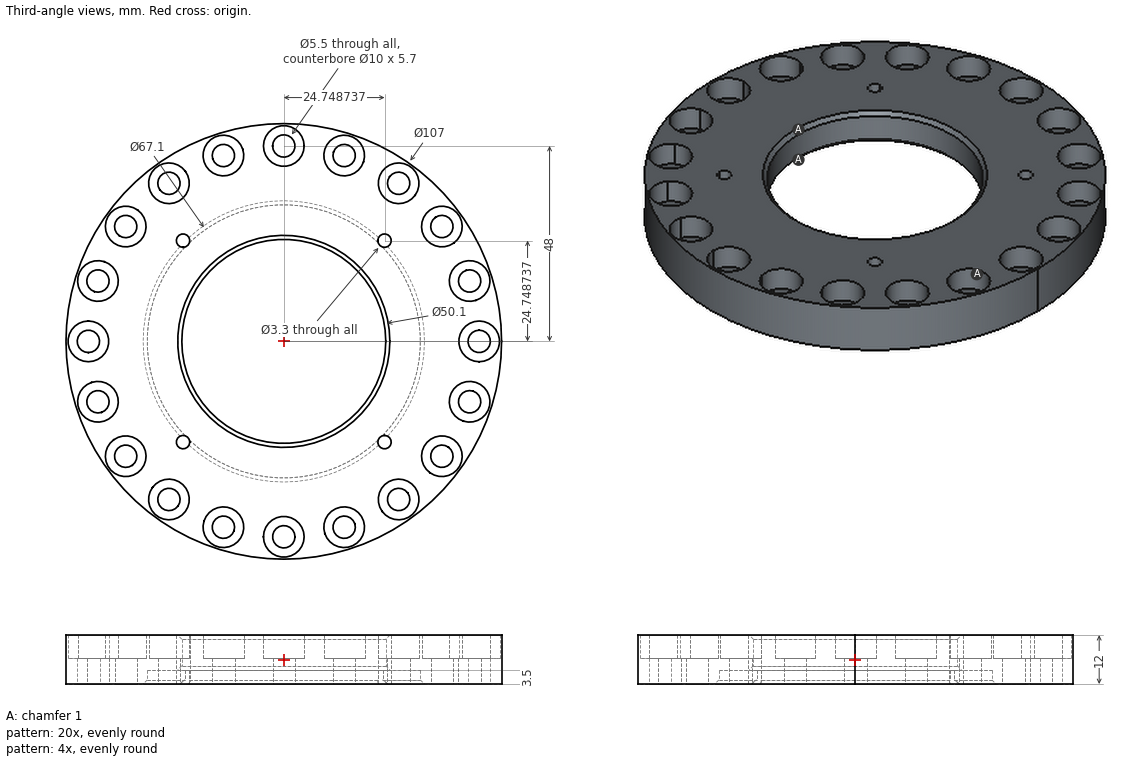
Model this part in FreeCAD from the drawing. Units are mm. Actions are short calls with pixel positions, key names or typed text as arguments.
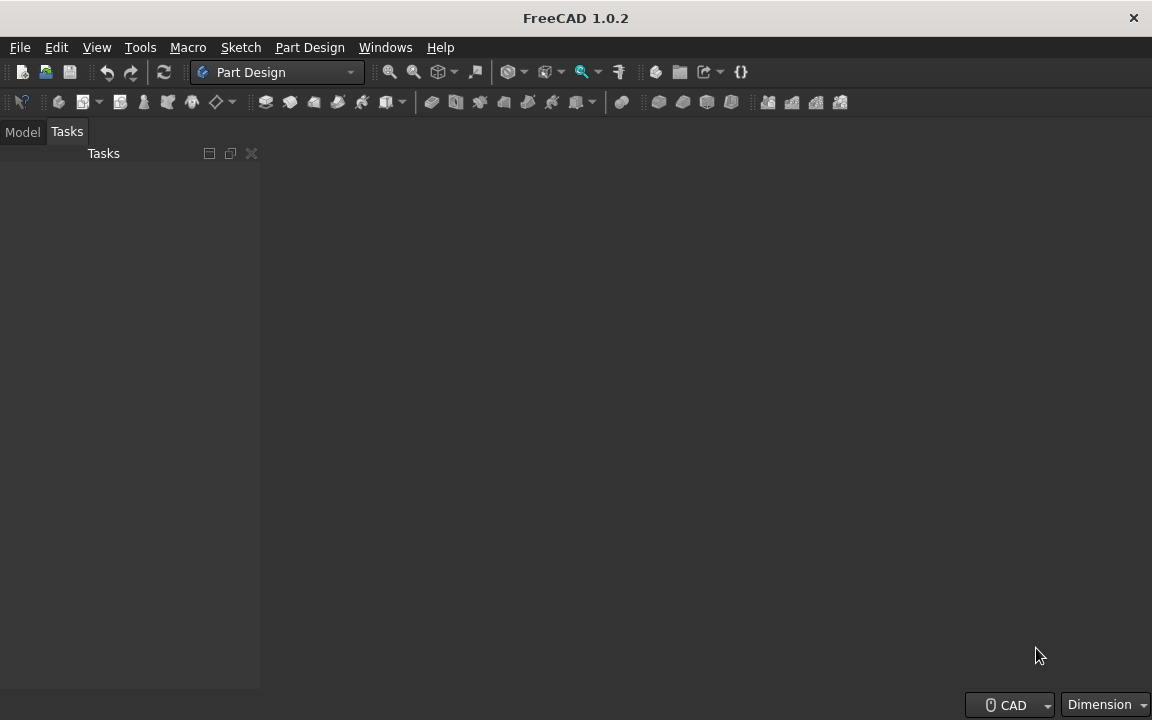
click(22, 72)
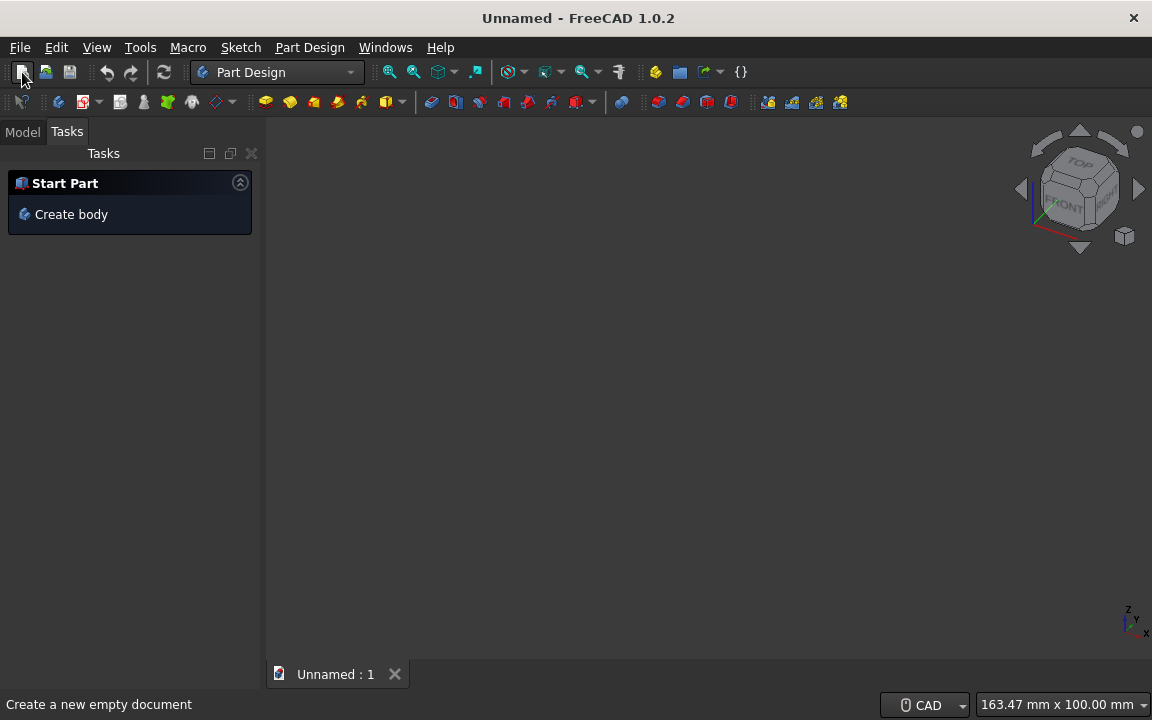
click(84, 102)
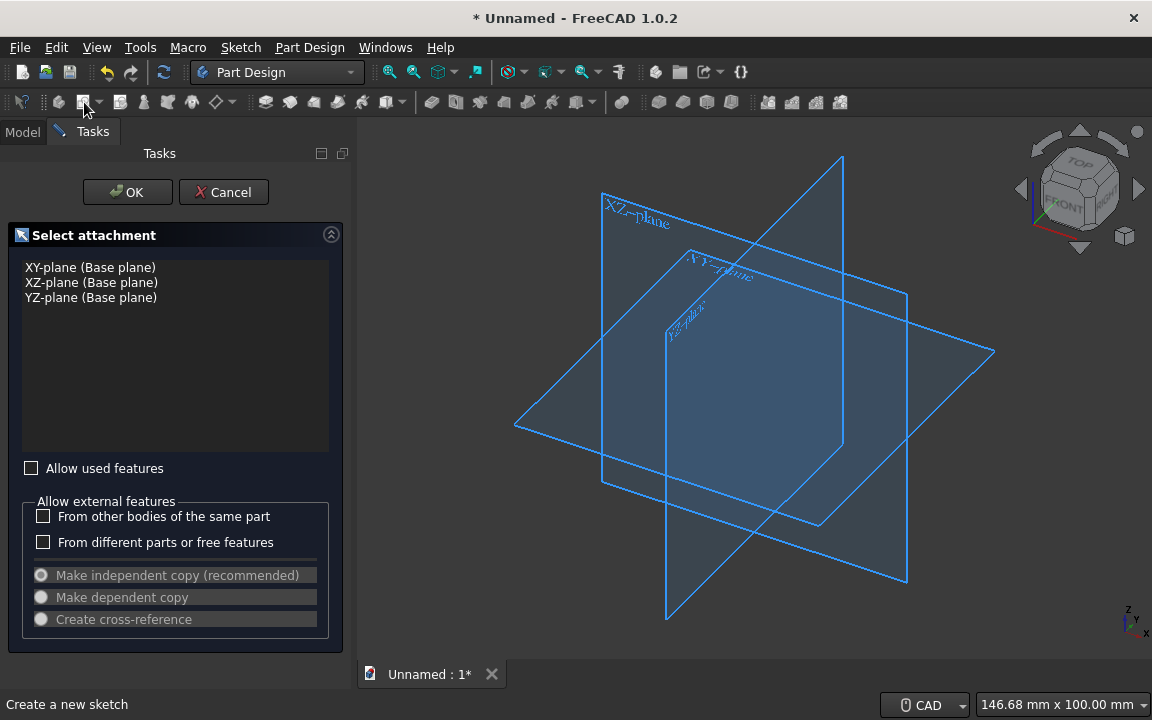
click(82, 268)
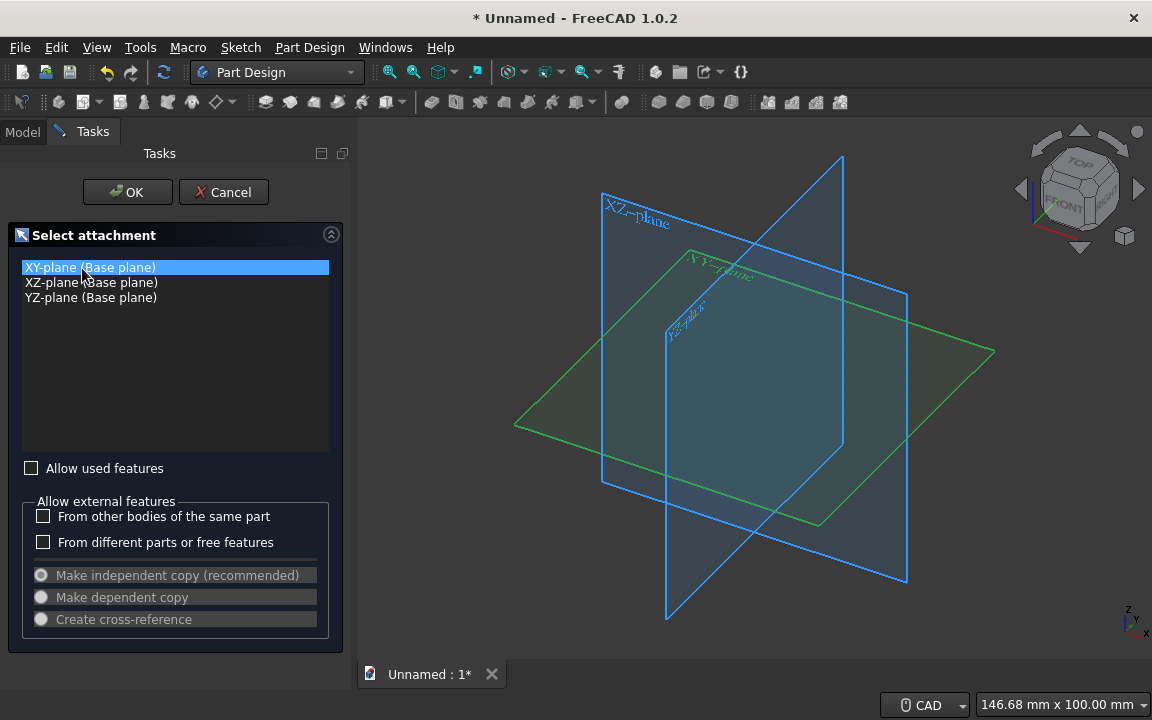
click(128, 192)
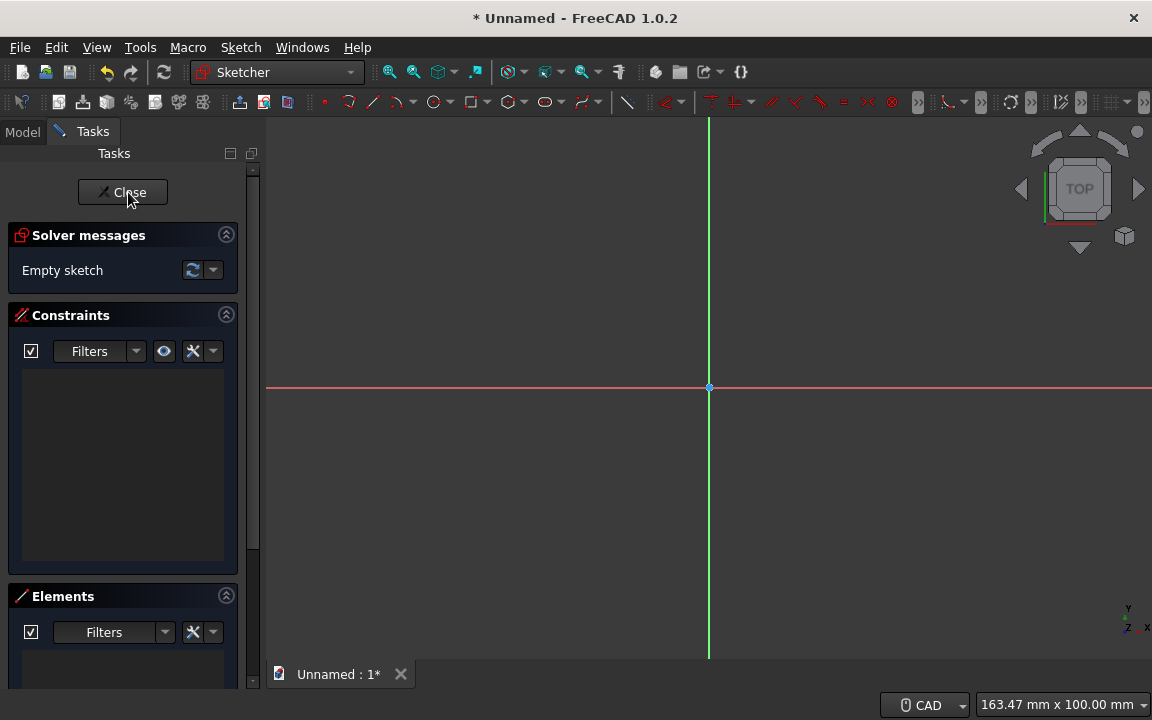
scroll(557, 388, down, 3)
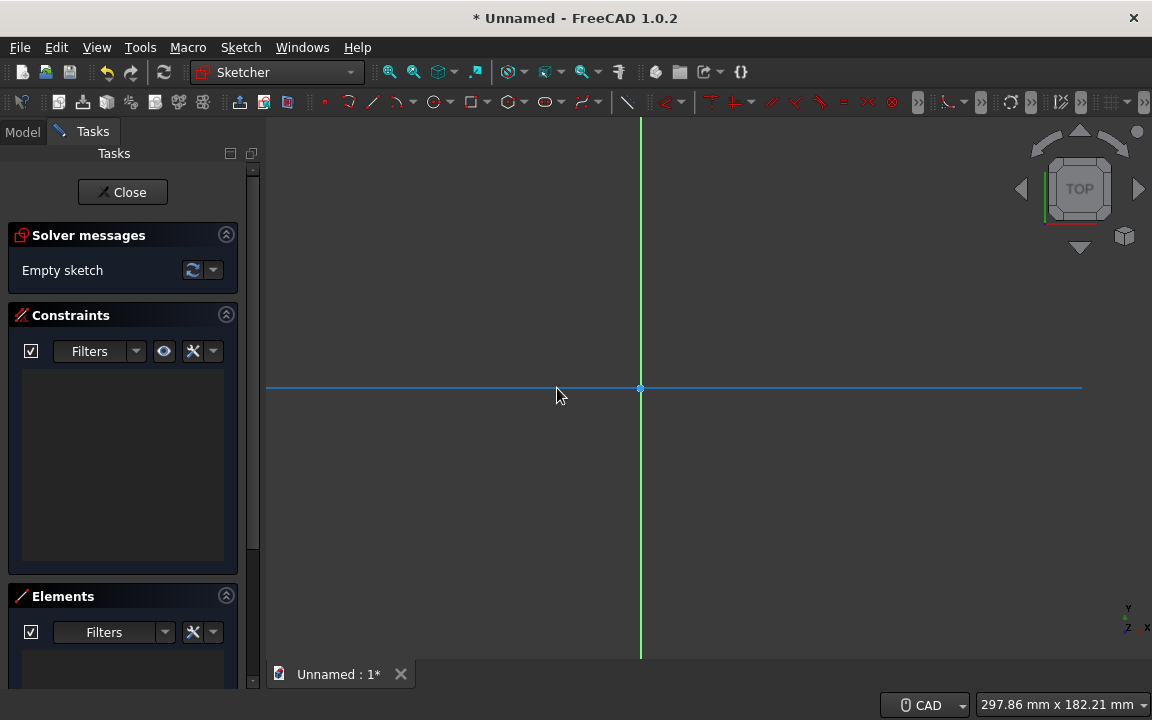
click(434, 102)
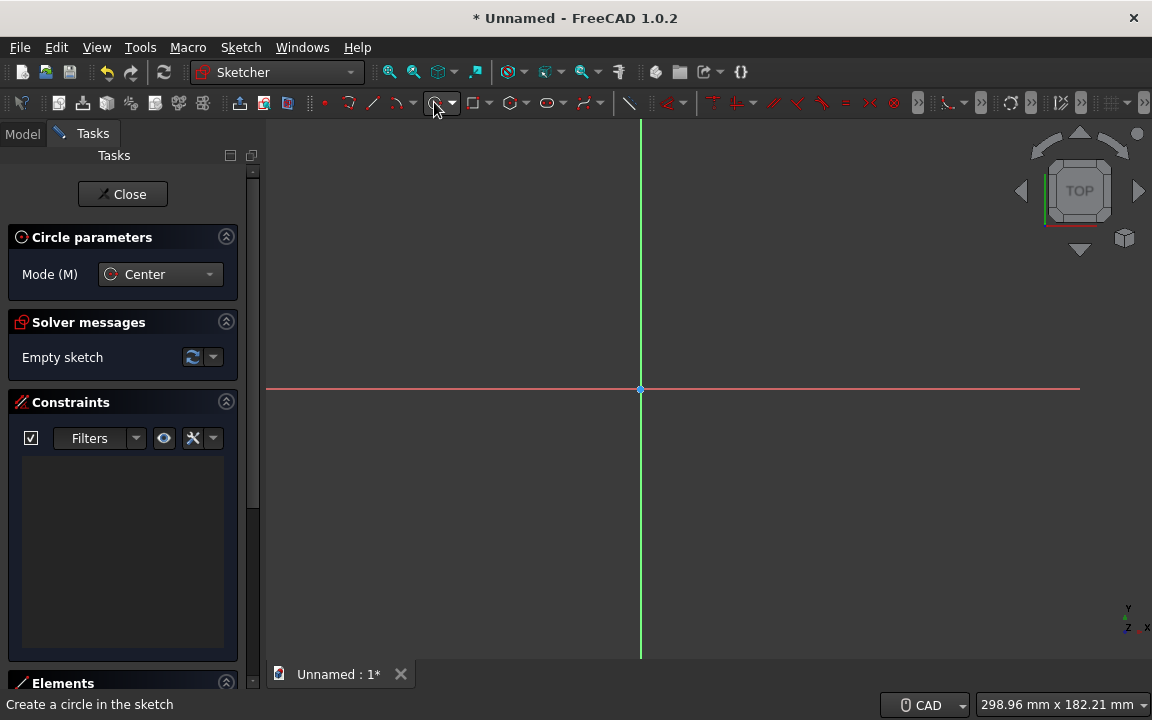
click(641, 389)
click(753, 277)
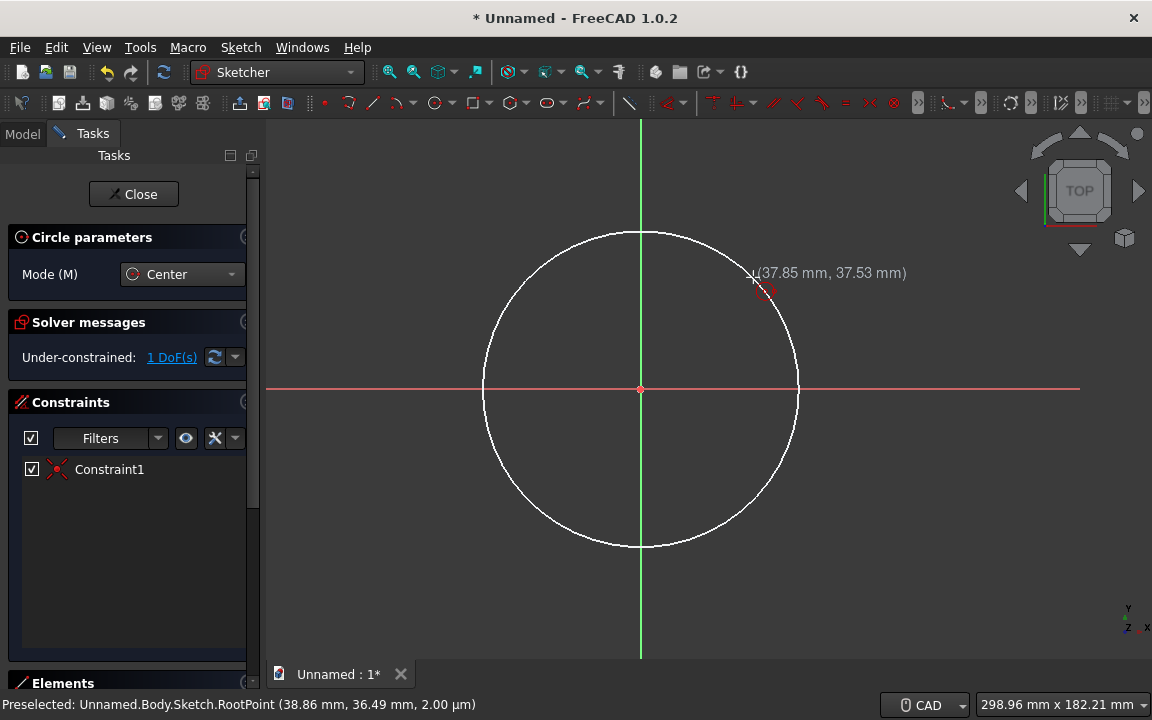
click(641, 389)
click(693, 337)
key(Escape)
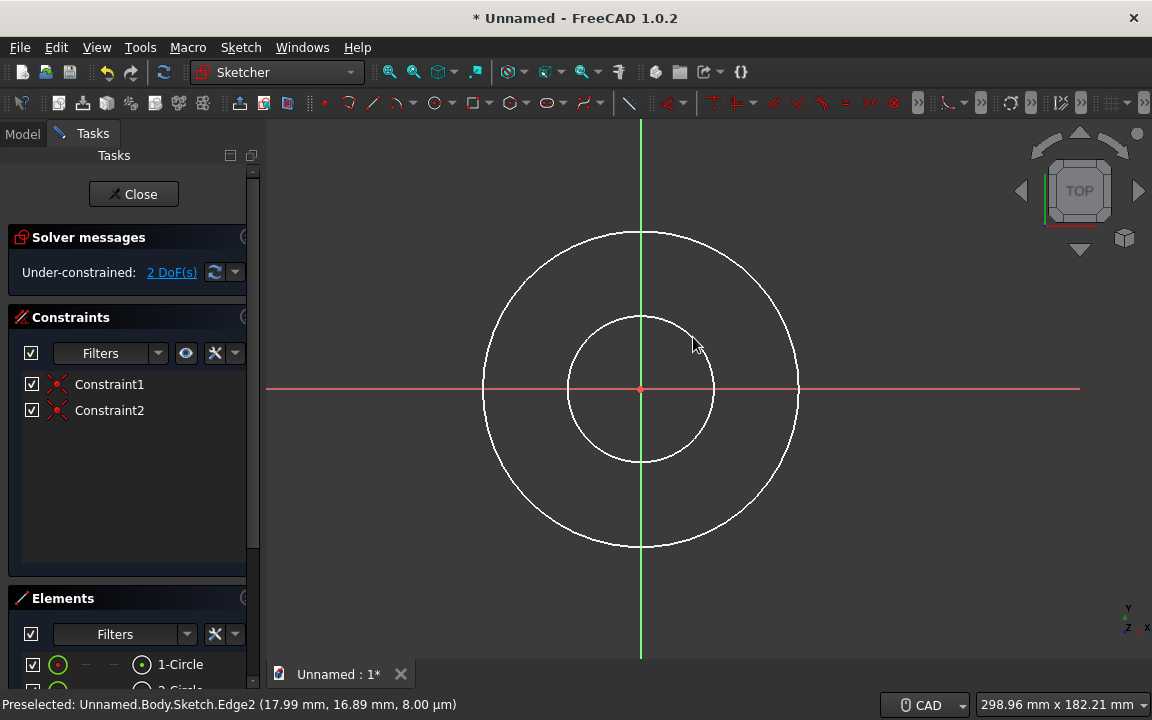
click(668, 104)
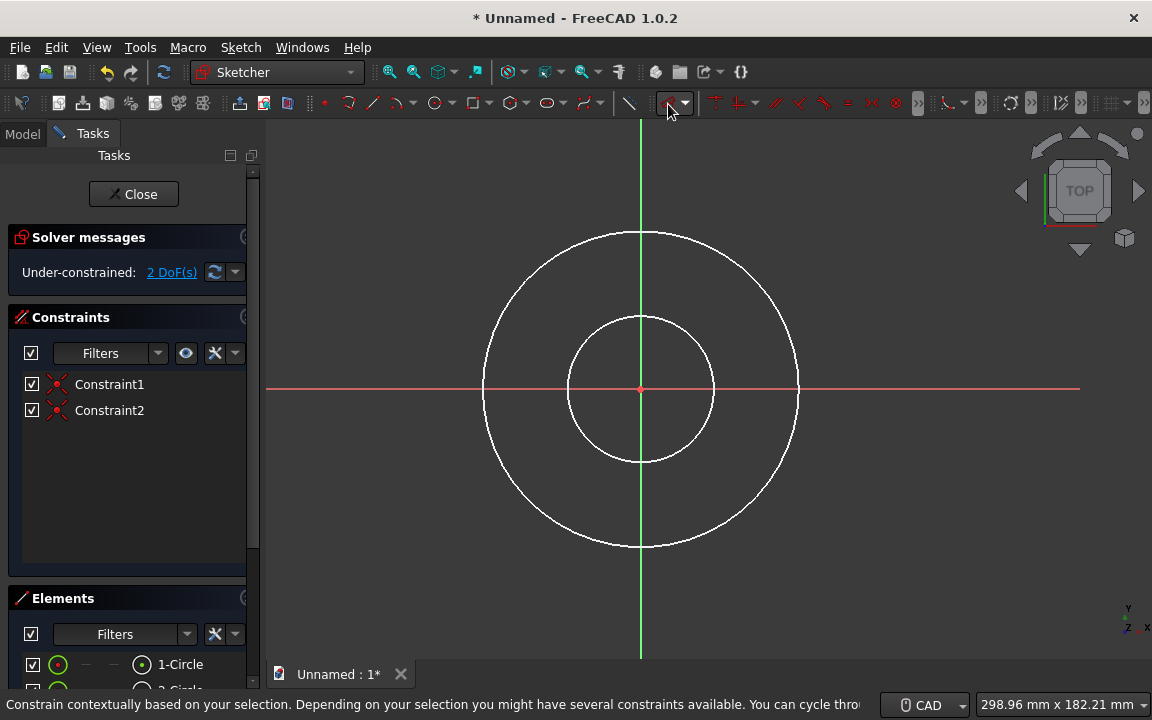
click(752, 277)
click(775, 254)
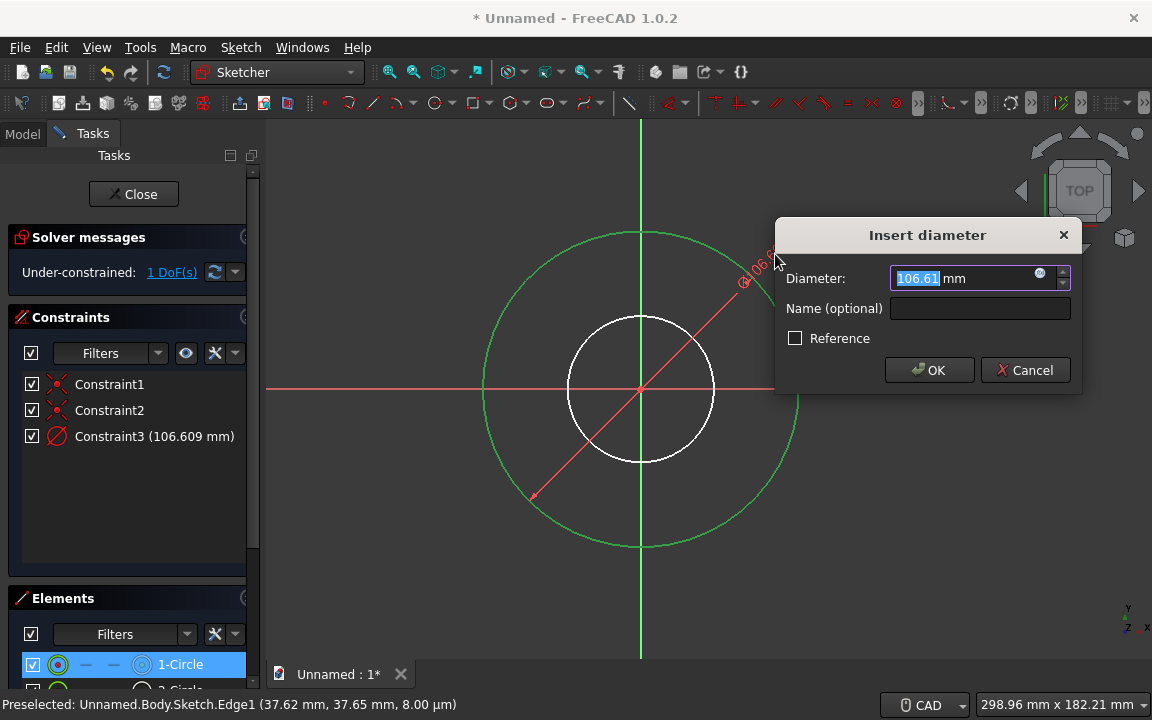
text(107)
key(Return)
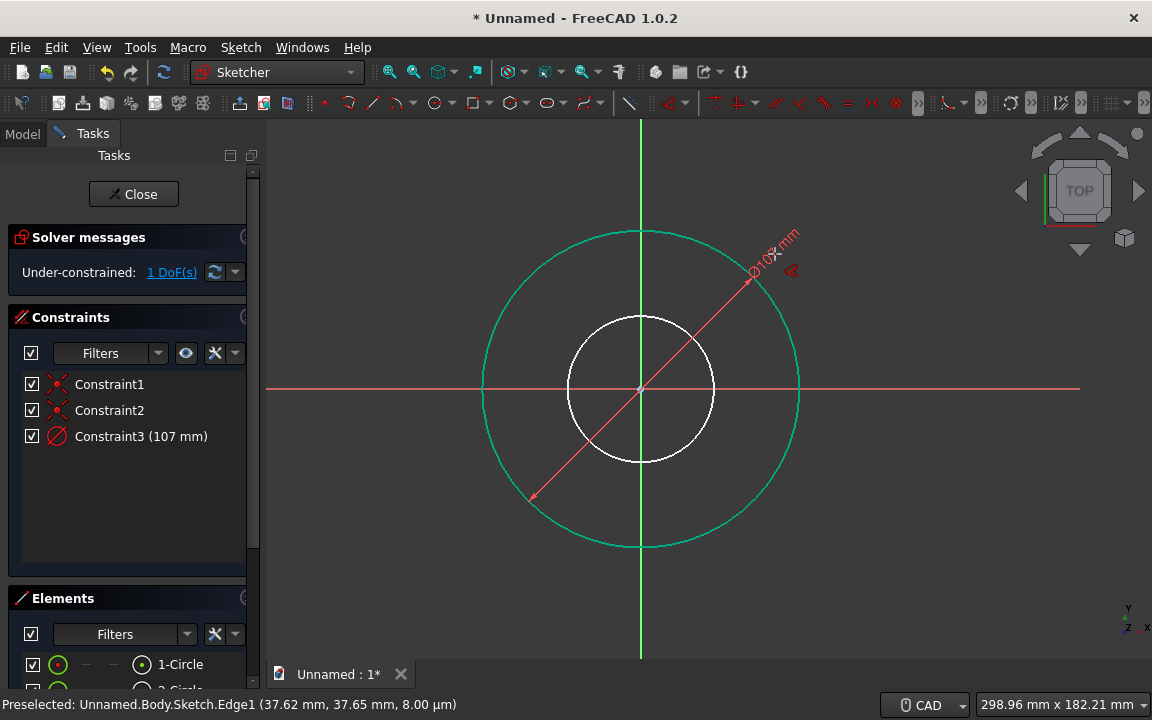
click(692, 337)
click(714, 314)